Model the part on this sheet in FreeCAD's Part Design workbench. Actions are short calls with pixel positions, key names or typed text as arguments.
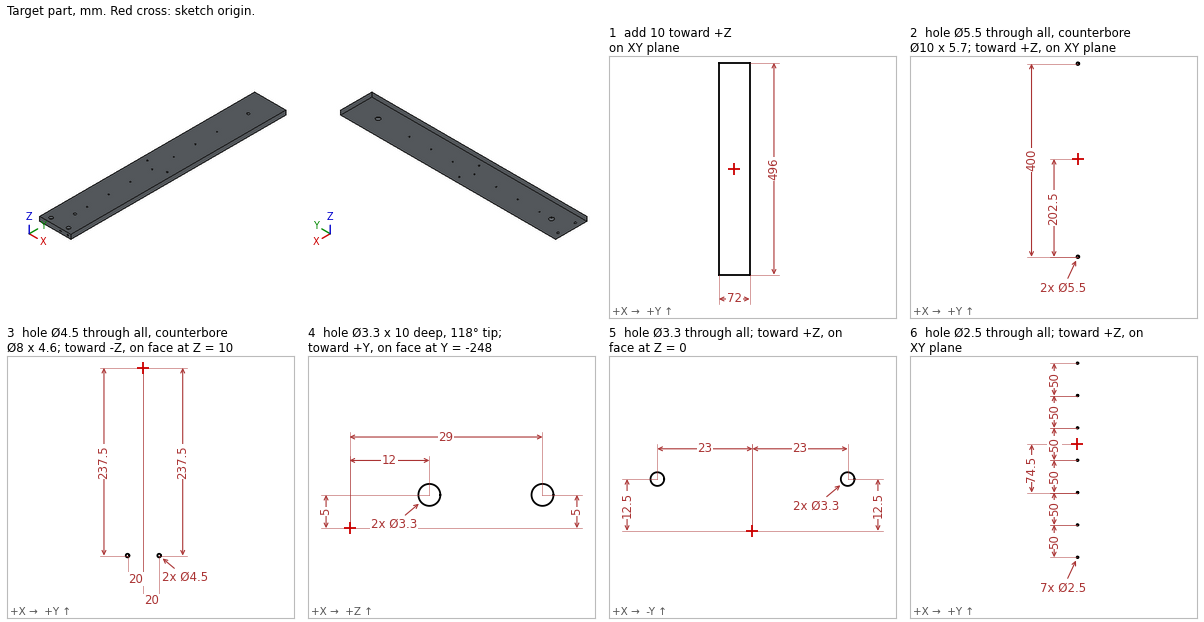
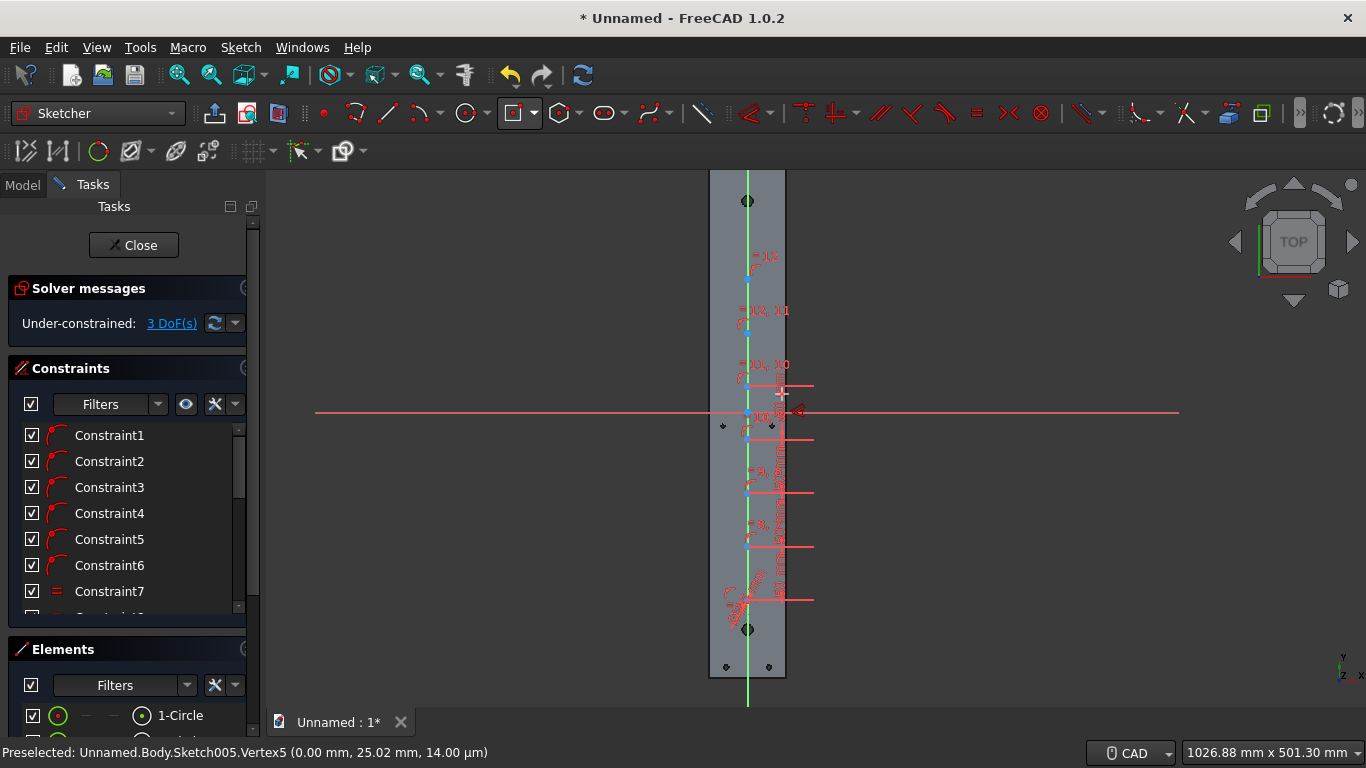
click(748, 386)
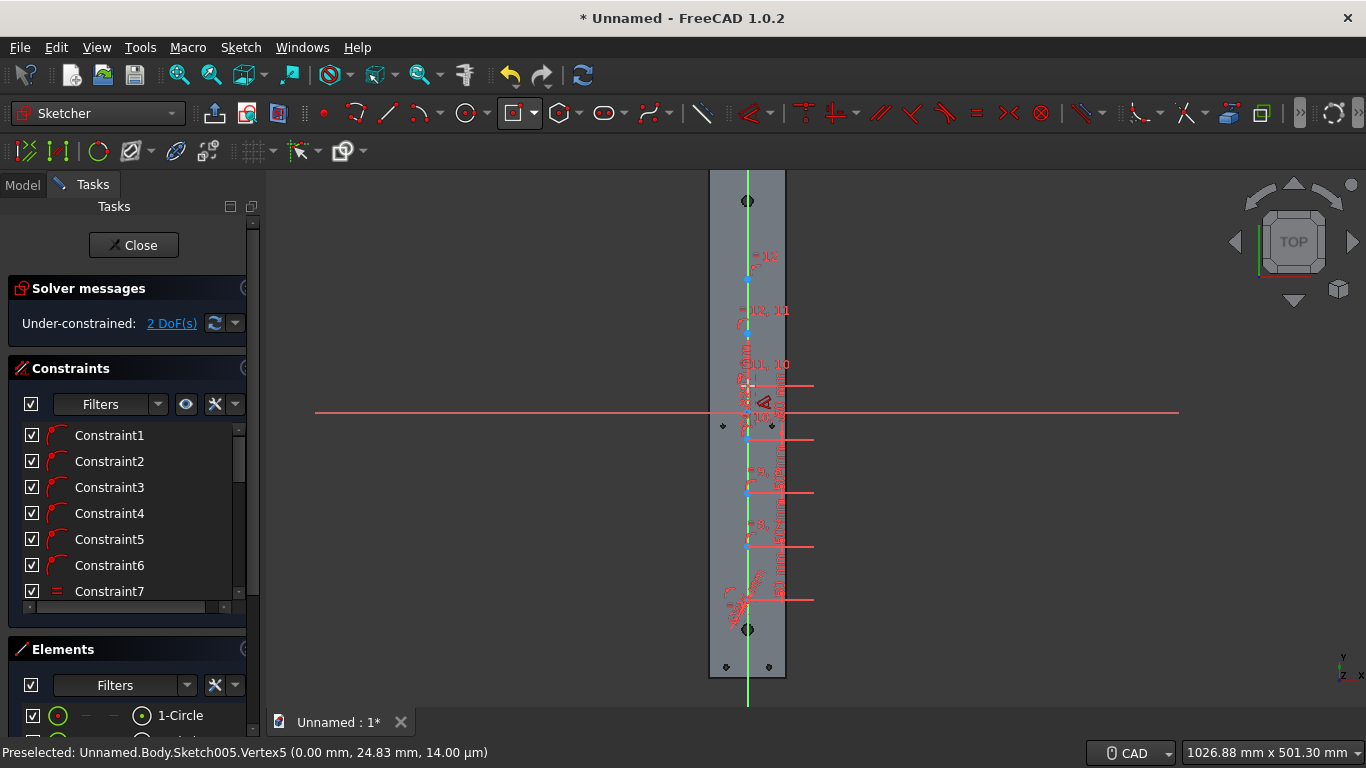
click(748, 333)
click(782, 360)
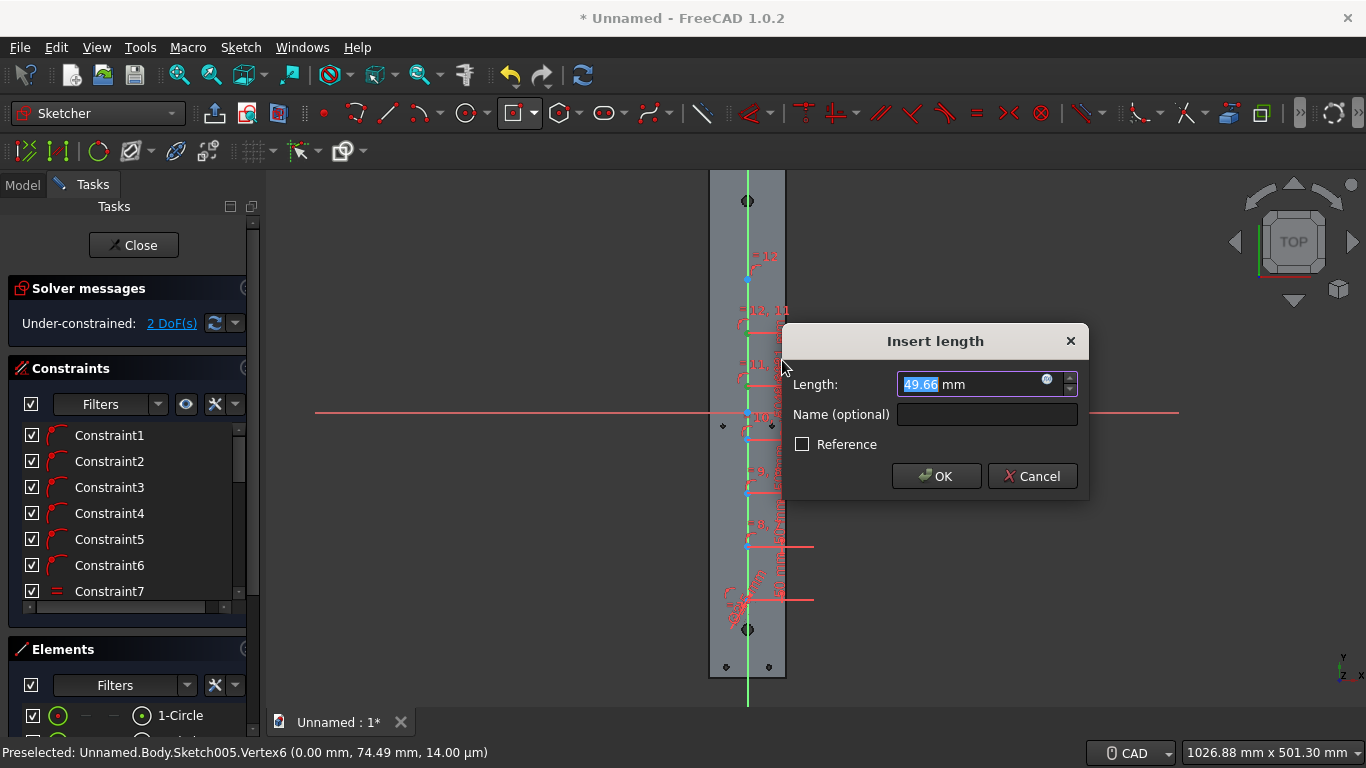
text(50)
key(Return)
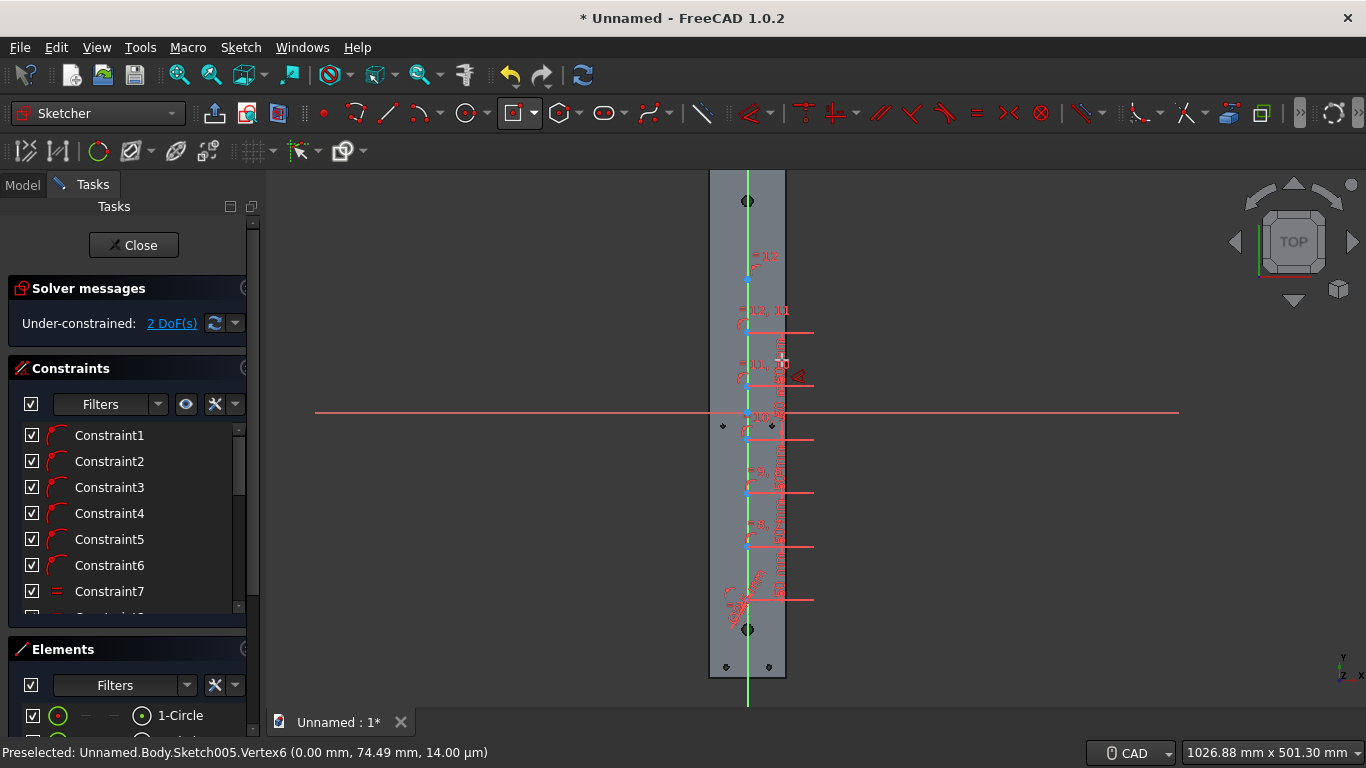
click(748, 333)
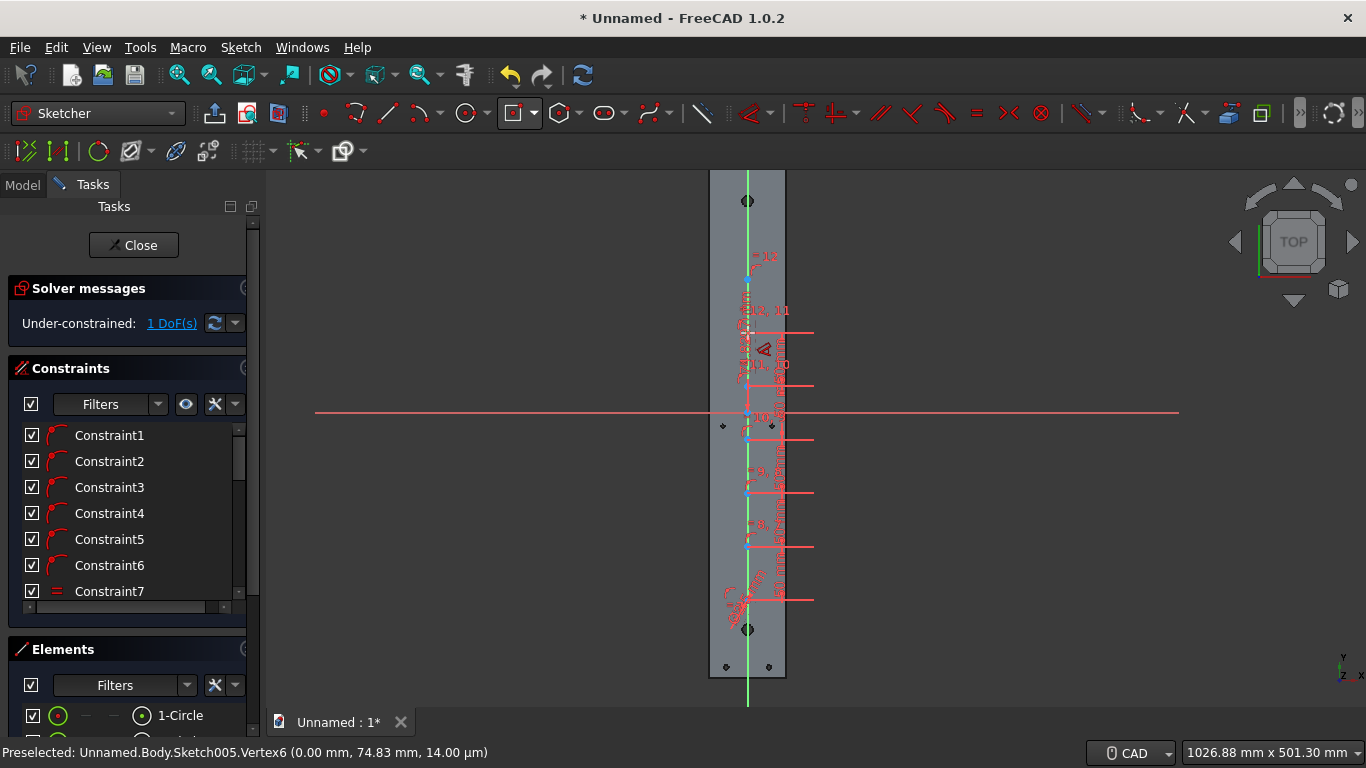
click(748, 279)
click(782, 306)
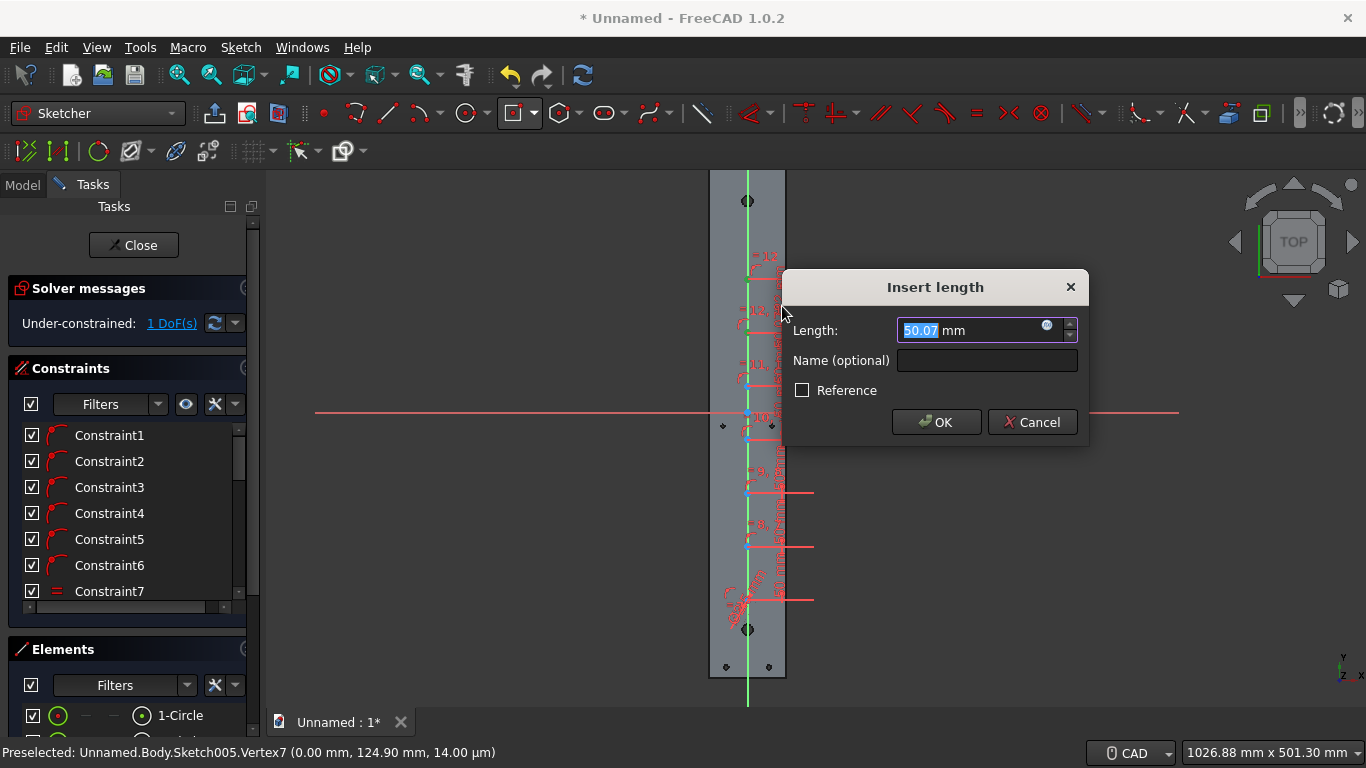
text(50)
key(Return)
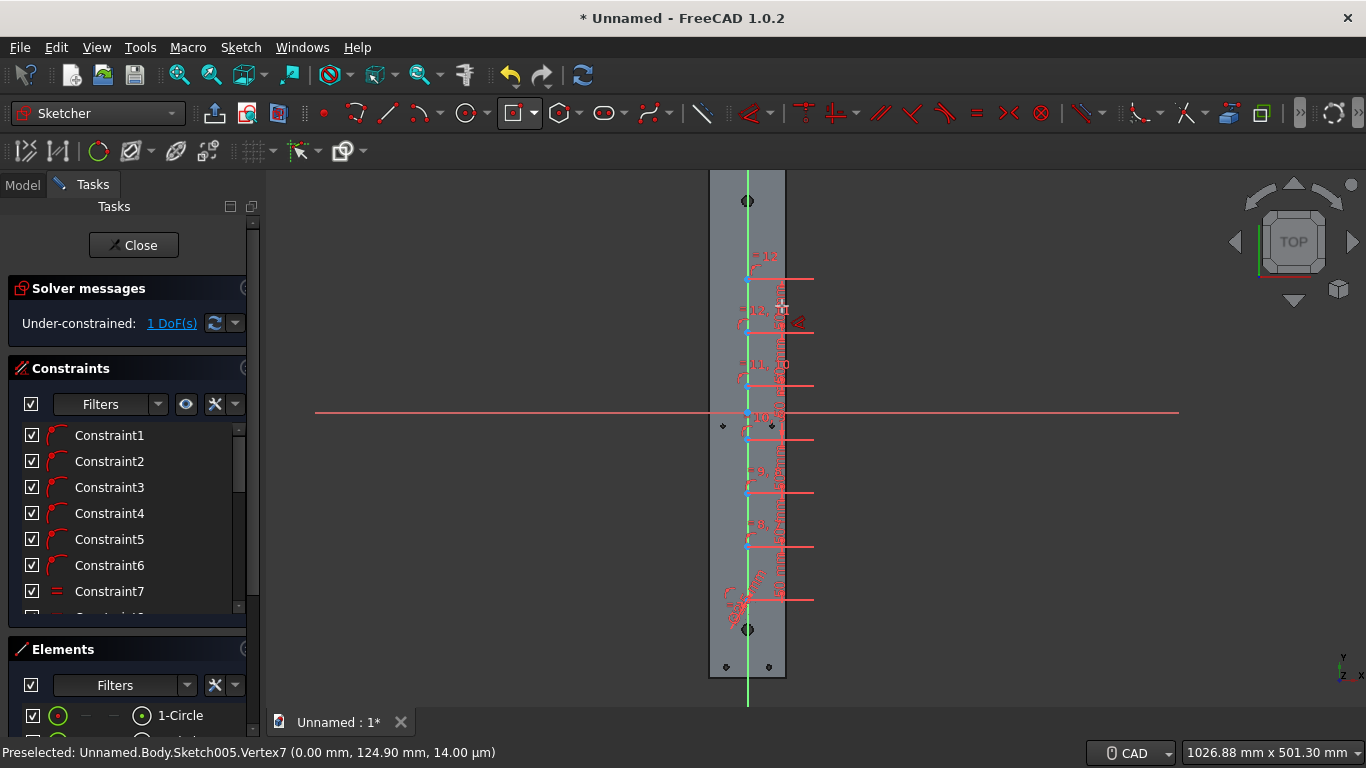
click(748, 493)
click(782, 435)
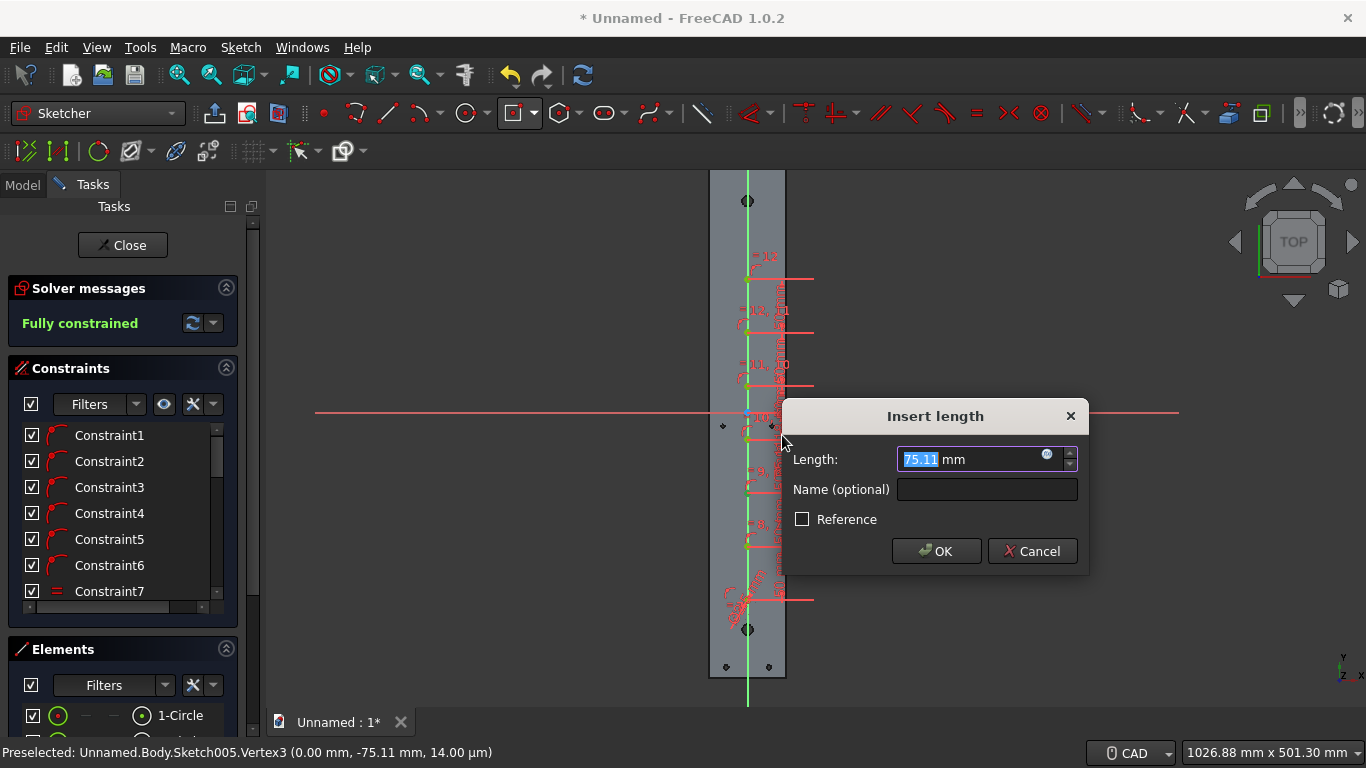
text(74.5)
key(Return)
key(Escape)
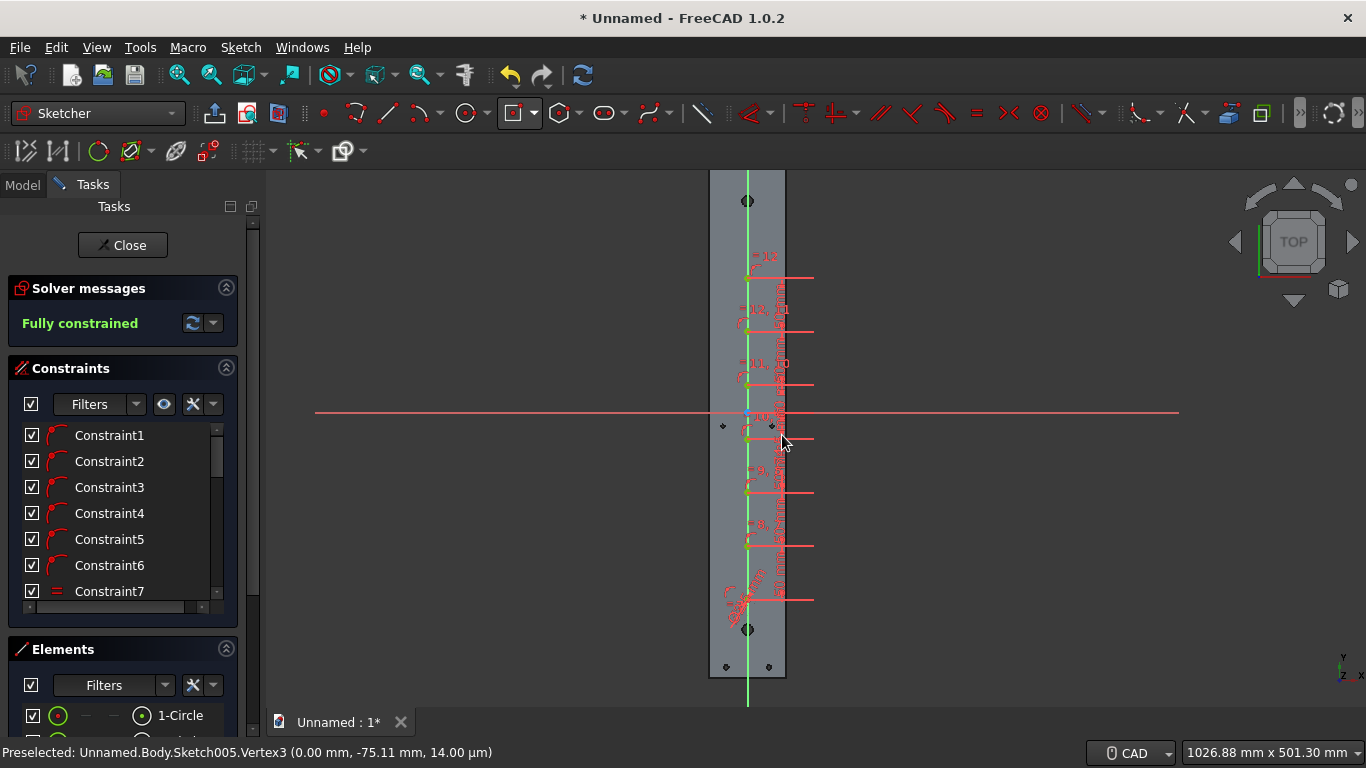
click(123, 245)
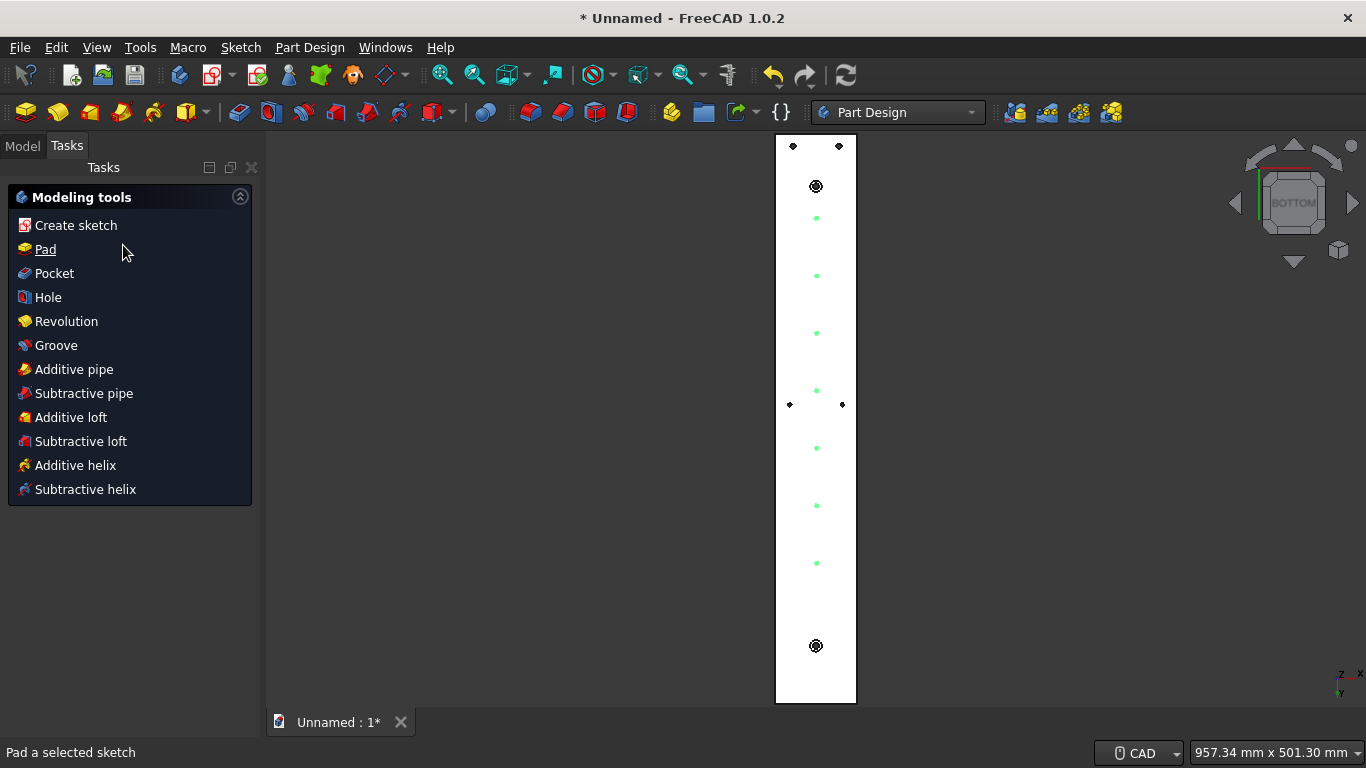
click(272, 112)